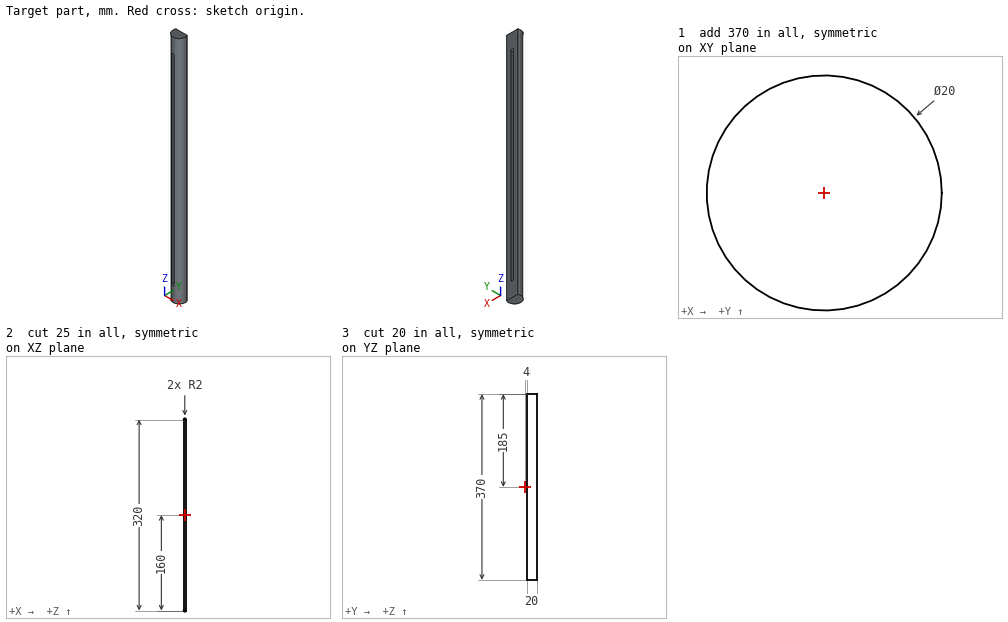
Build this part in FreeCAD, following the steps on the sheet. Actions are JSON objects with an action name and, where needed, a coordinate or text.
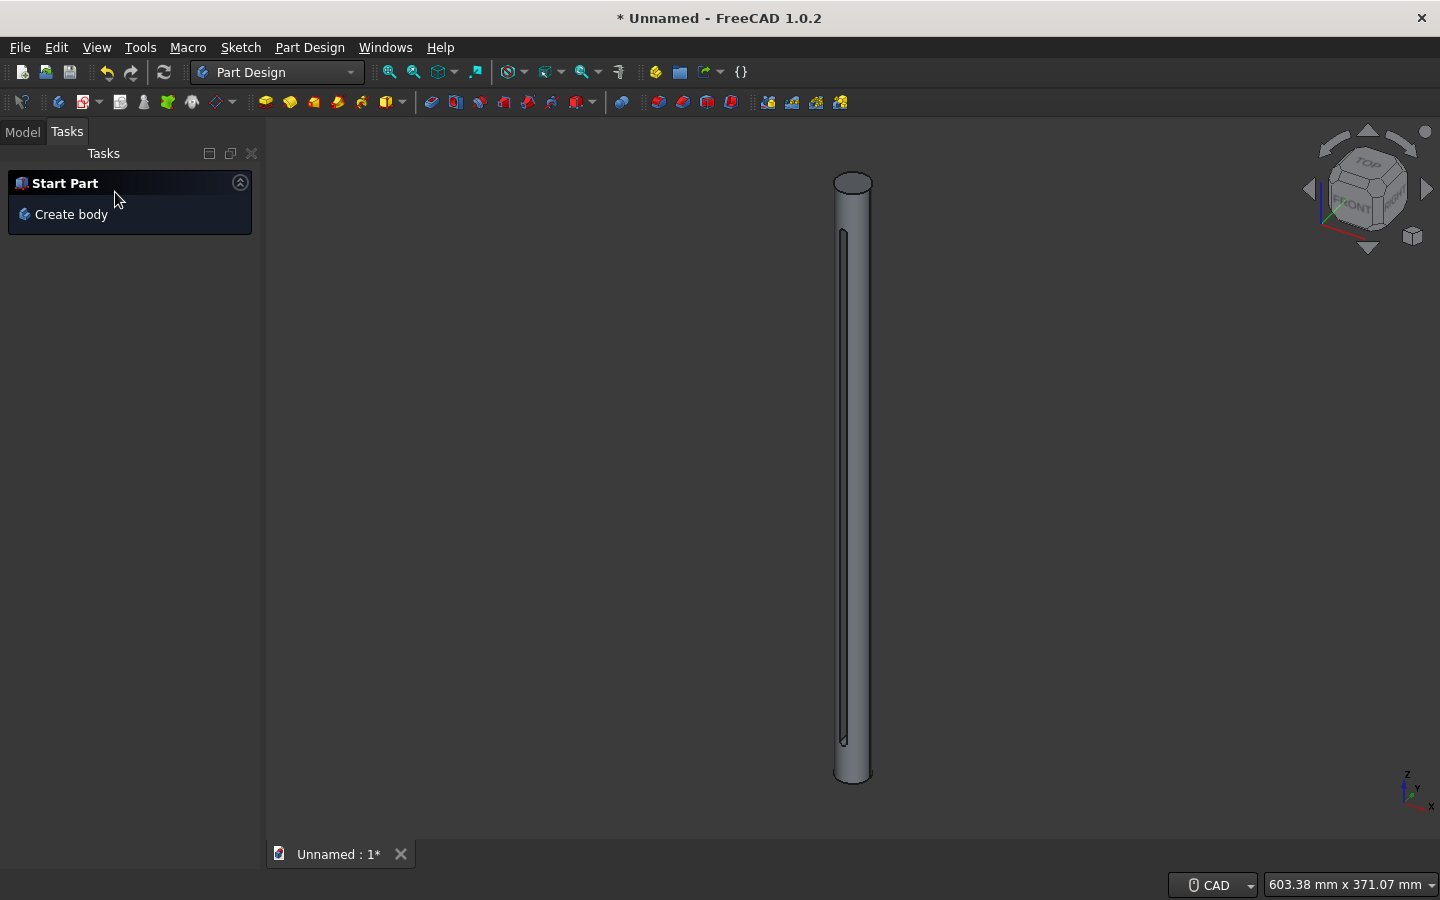
{"action": "left_click", "coordinate": [84, 102]}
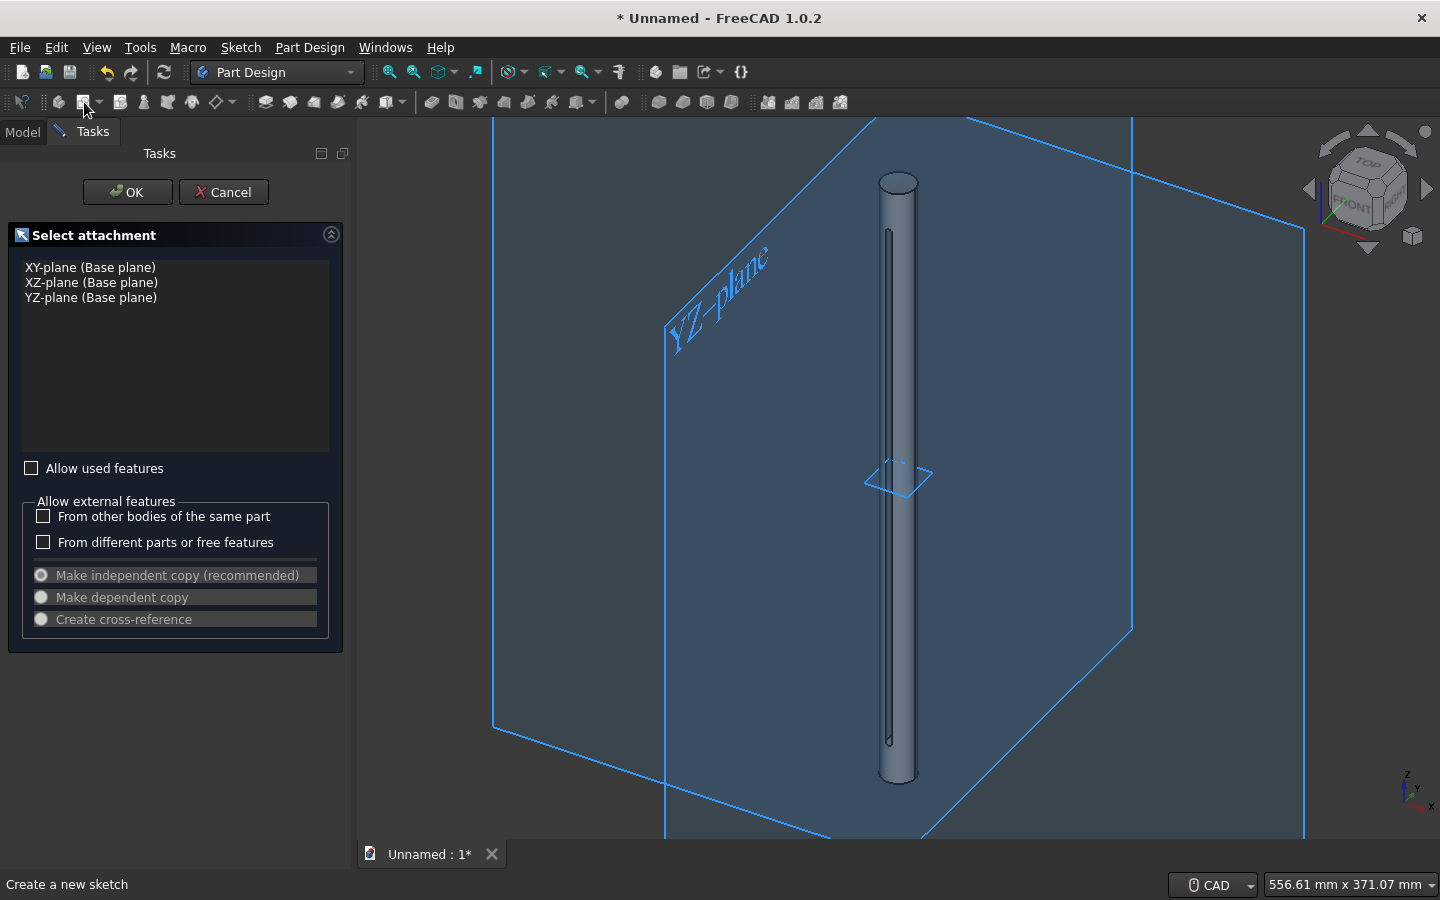
{"action": "left_click", "coordinate": [82, 298]}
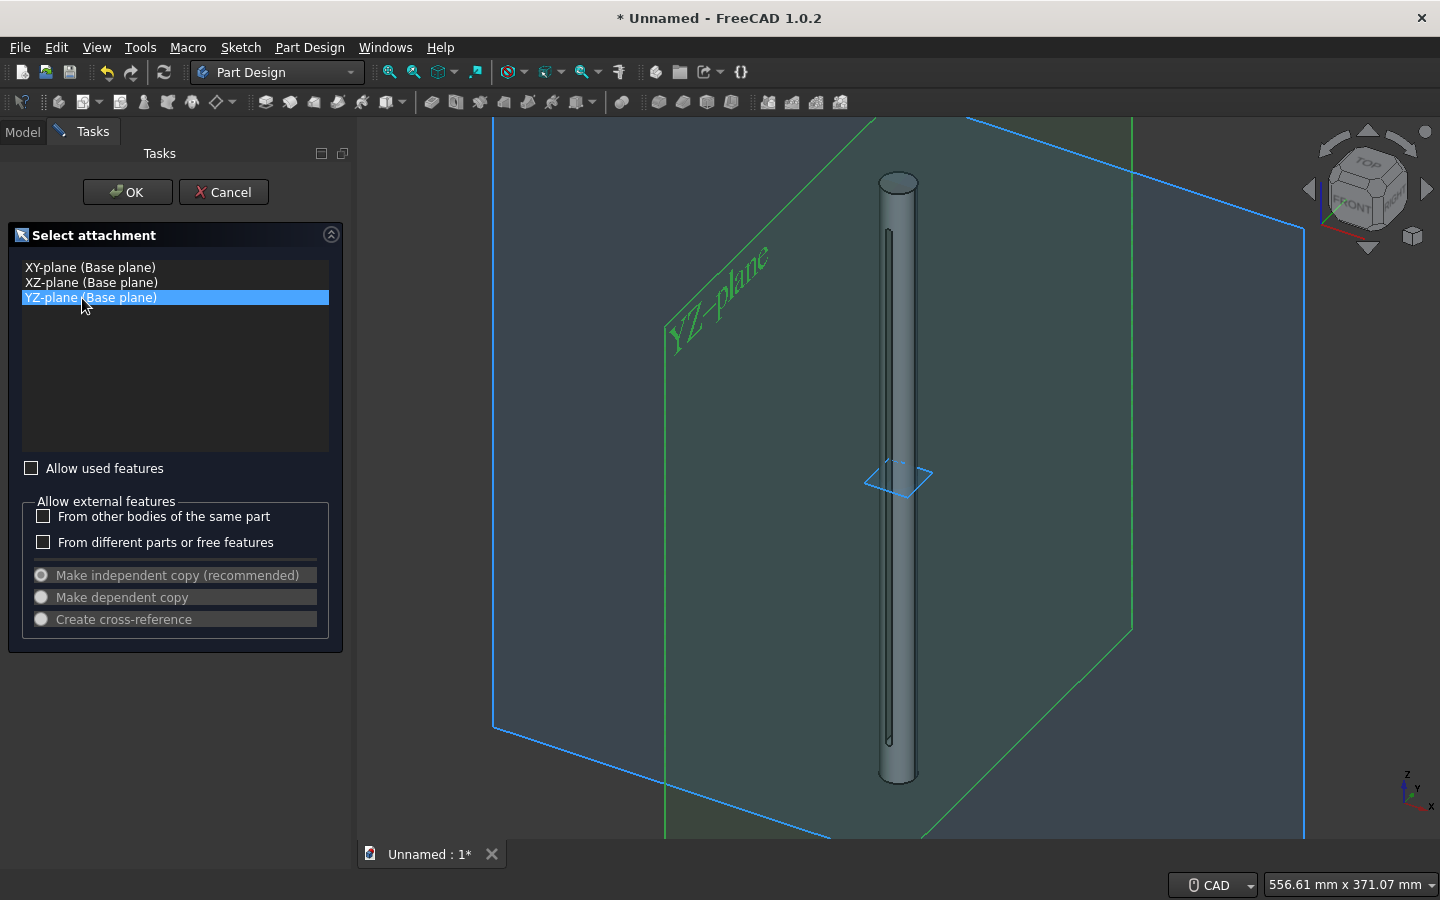
{"action": "left_click", "coordinate": [128, 192]}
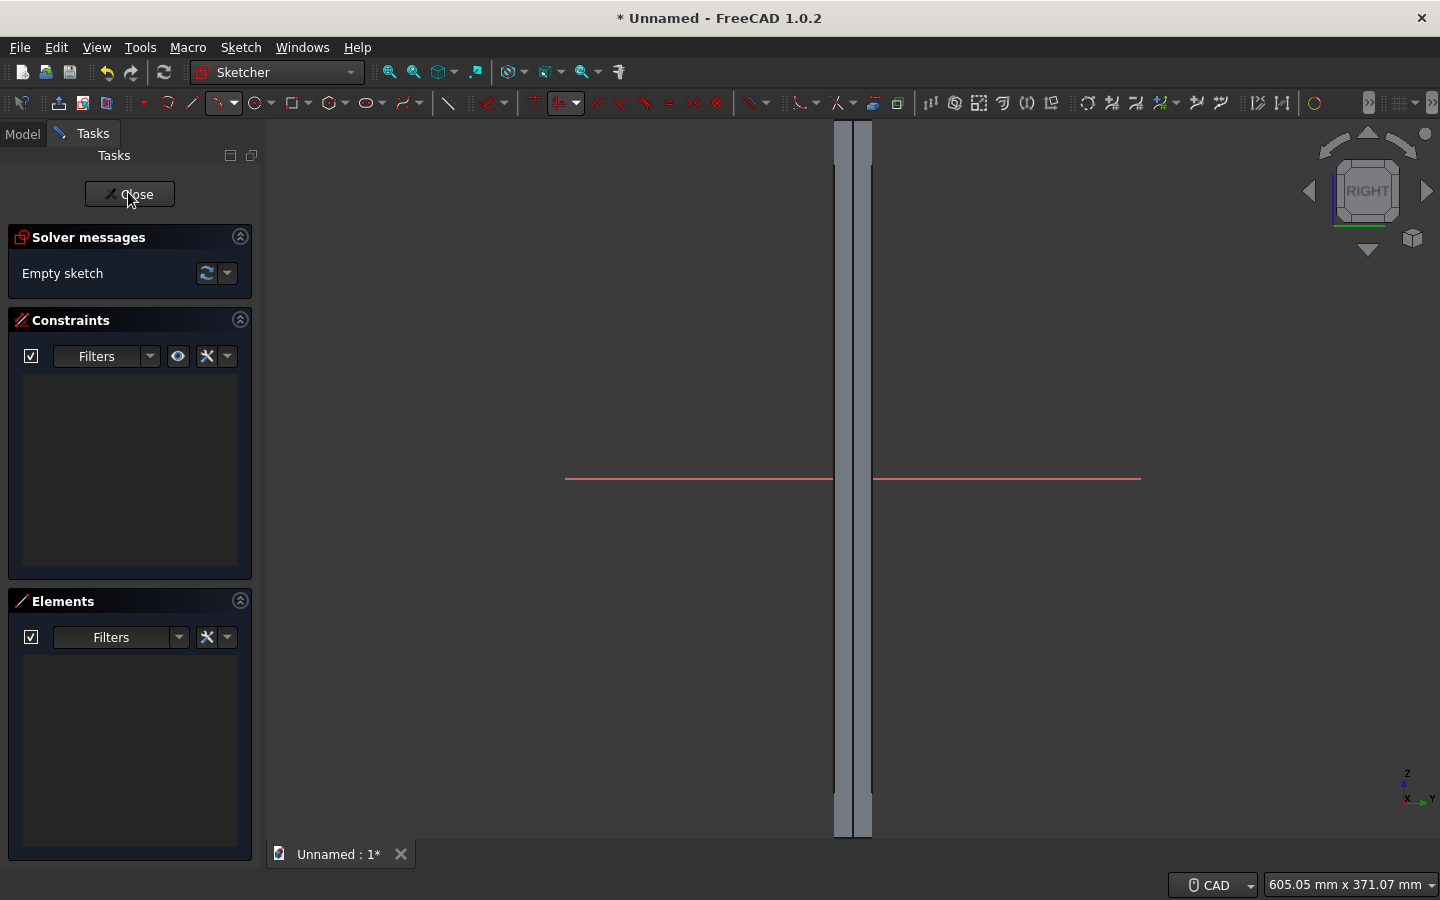
{"action": "left_click", "coordinate": [108, 104]}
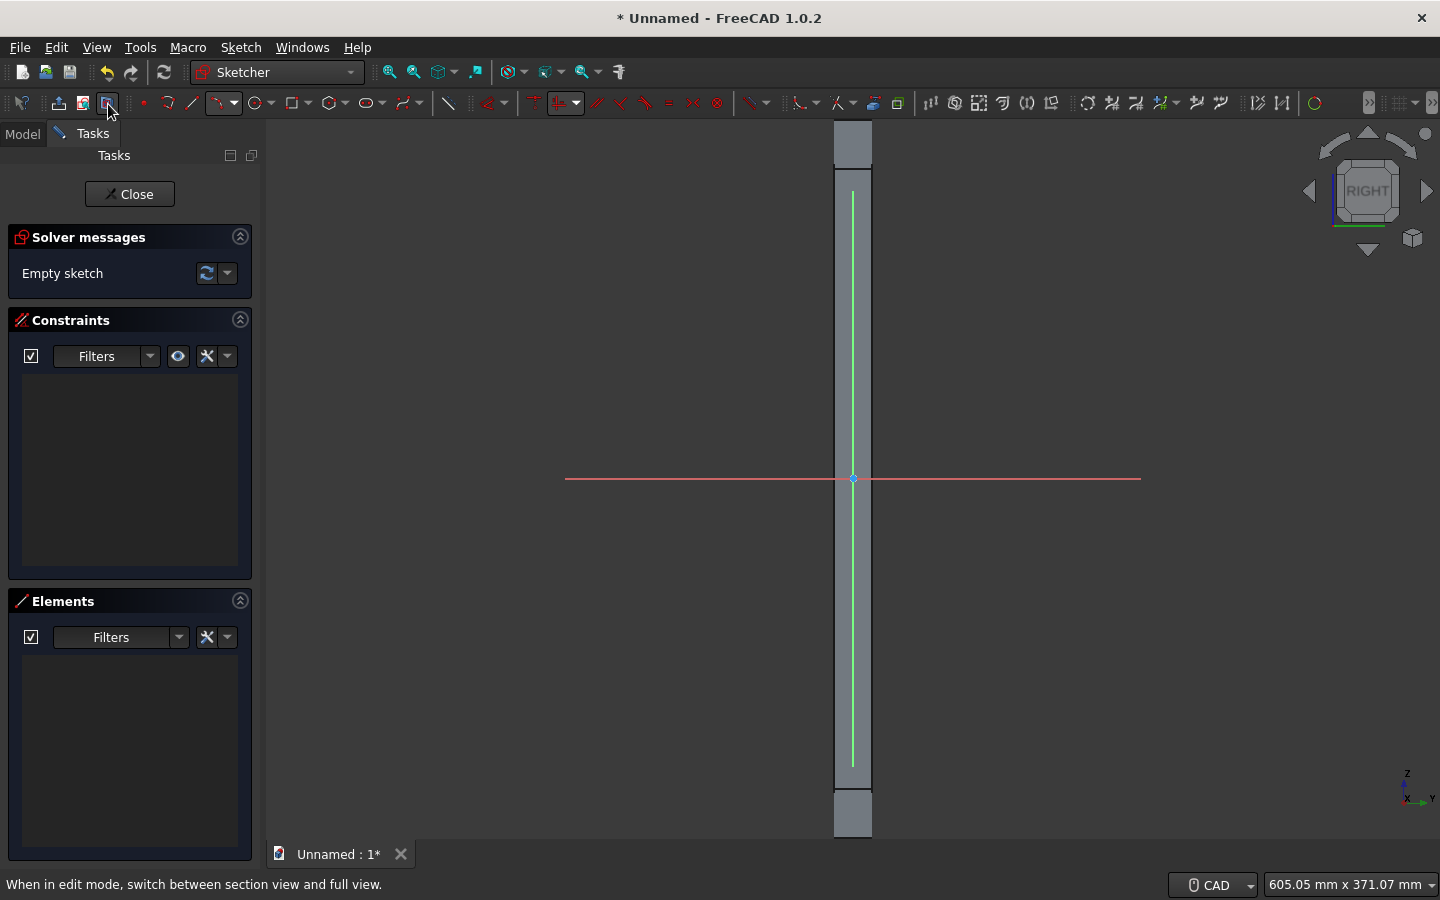
{"action": "scroll", "coordinate": [598, 479], "scroll_direction": "down", "scroll_amount": 2}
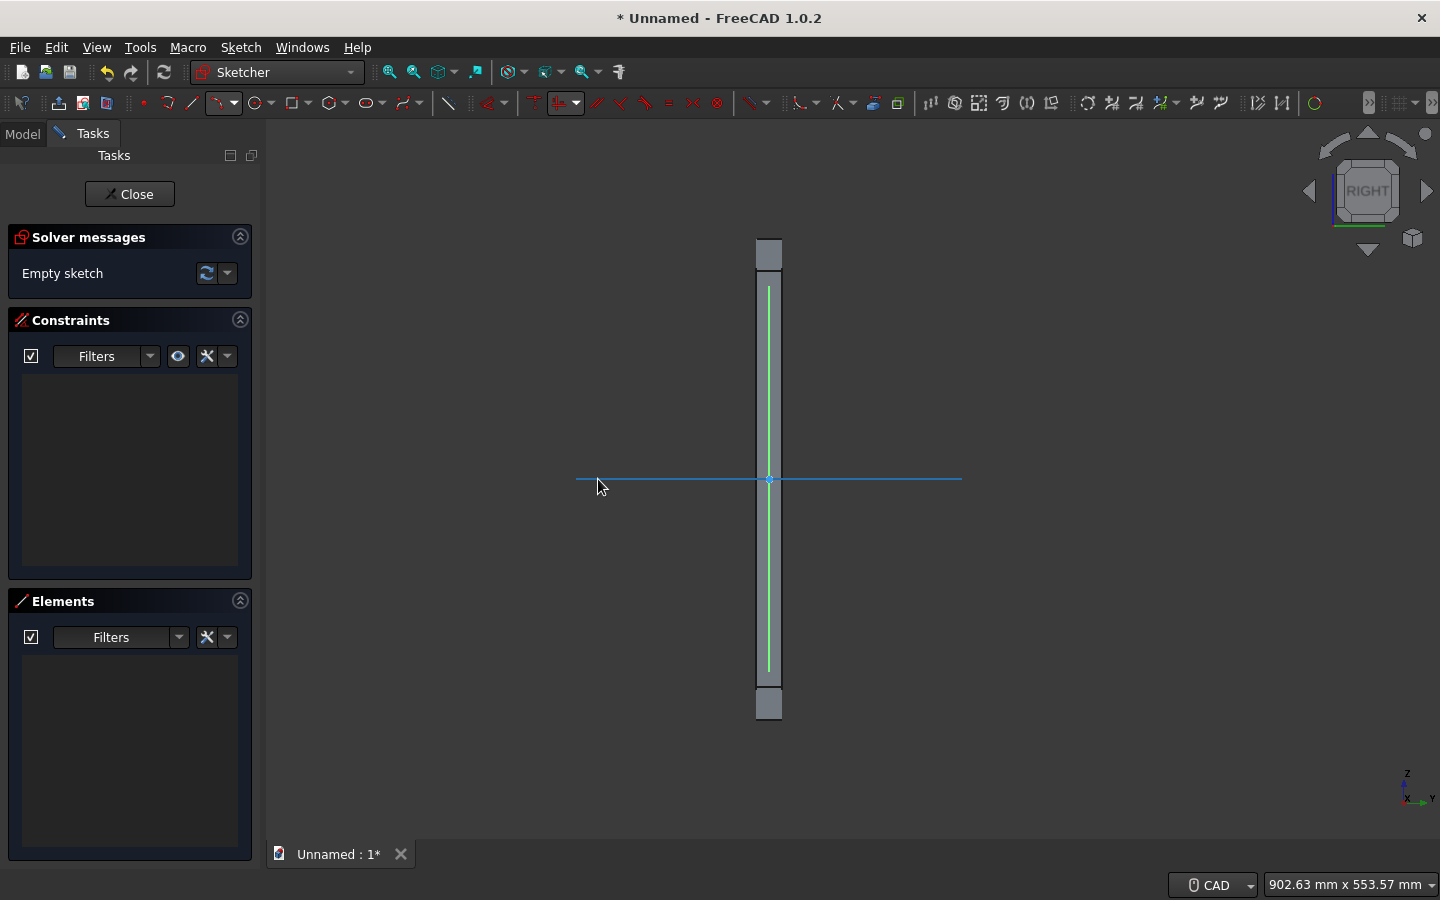
{"action": "left_click", "coordinate": [292, 104]}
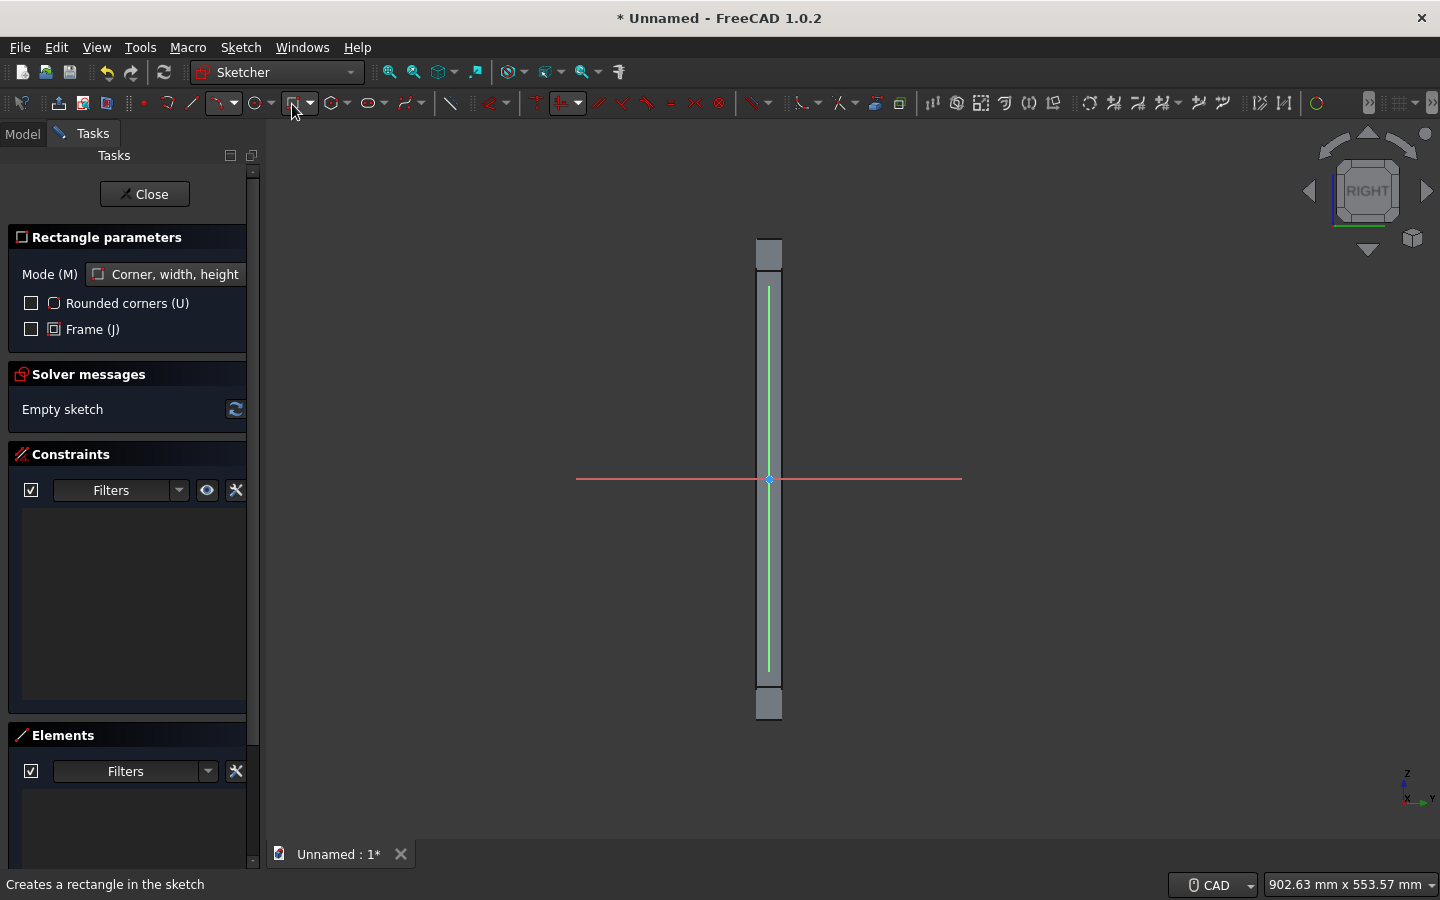
{"action": "scroll", "coordinate": [774, 239], "scroll_direction": "up", "scroll_amount": 6}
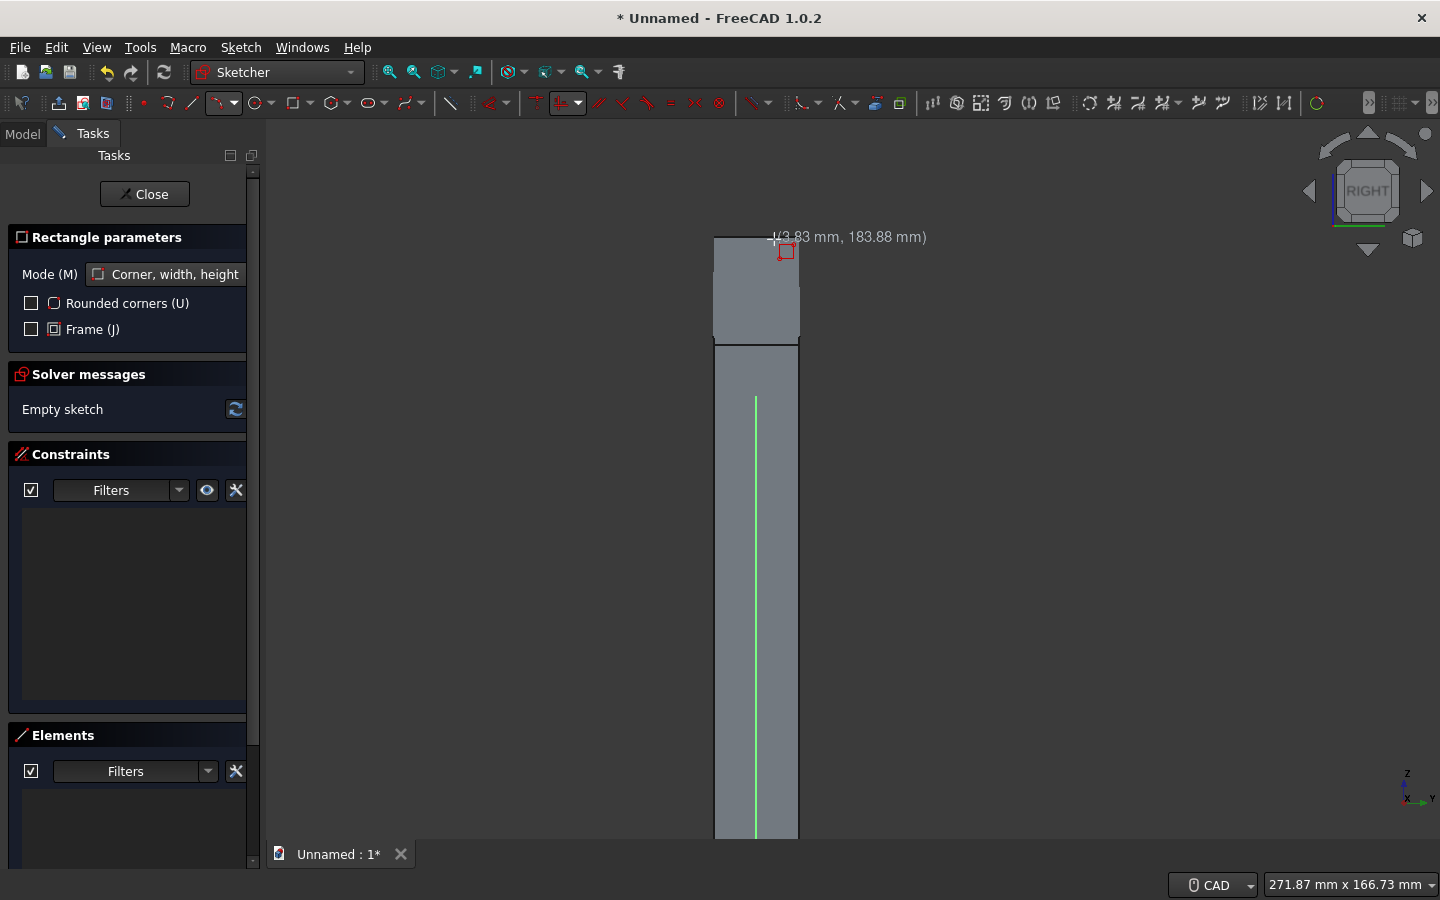
{"action": "left_click", "coordinate": [774, 237]}